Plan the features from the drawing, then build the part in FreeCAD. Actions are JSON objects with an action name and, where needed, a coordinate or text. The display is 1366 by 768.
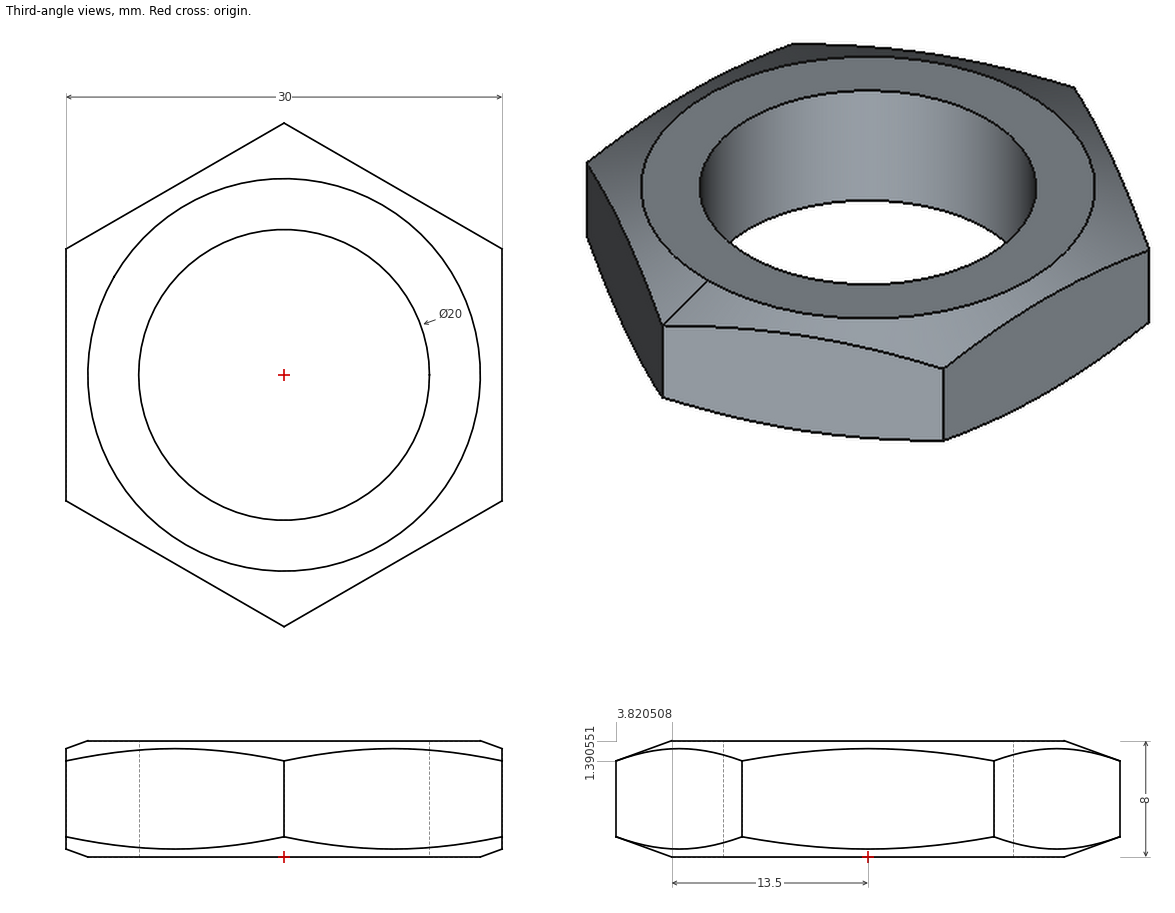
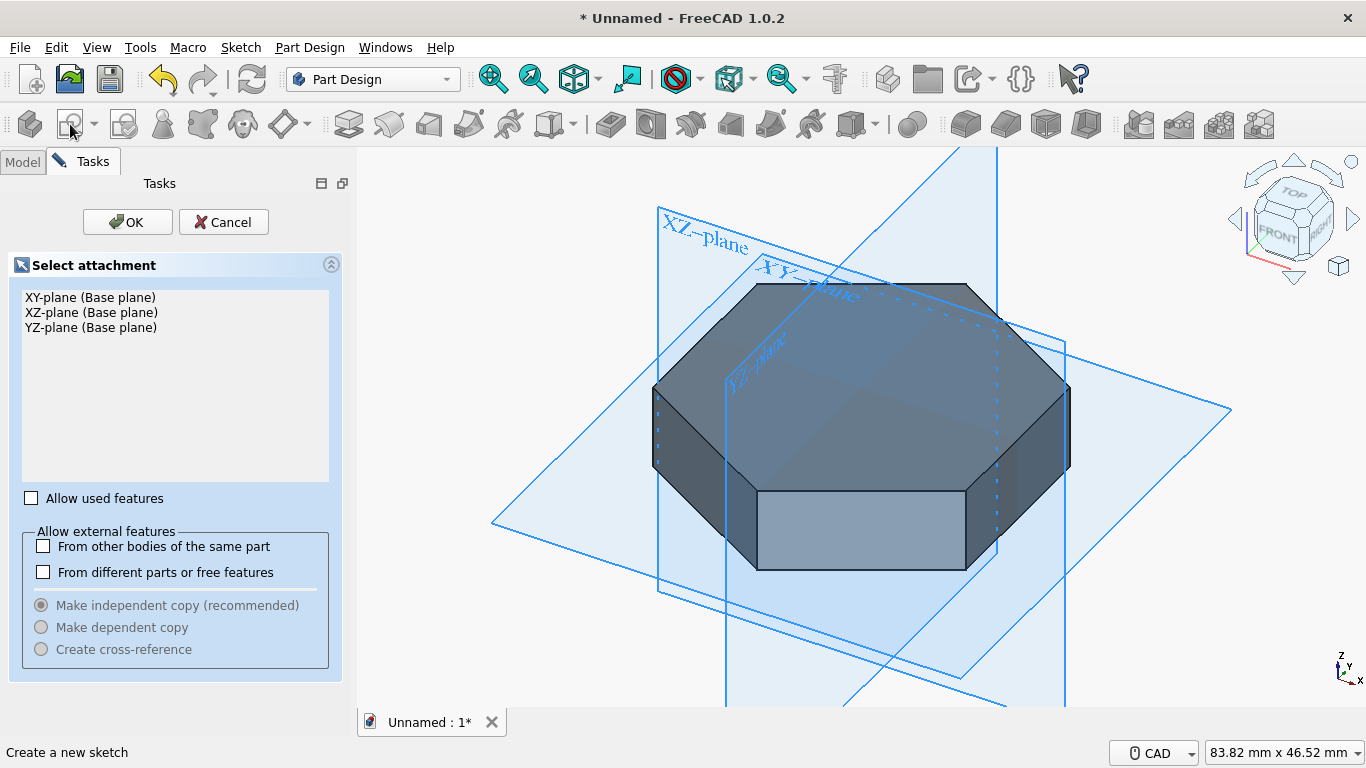
{"action": "left_click", "coordinate": [82, 328]}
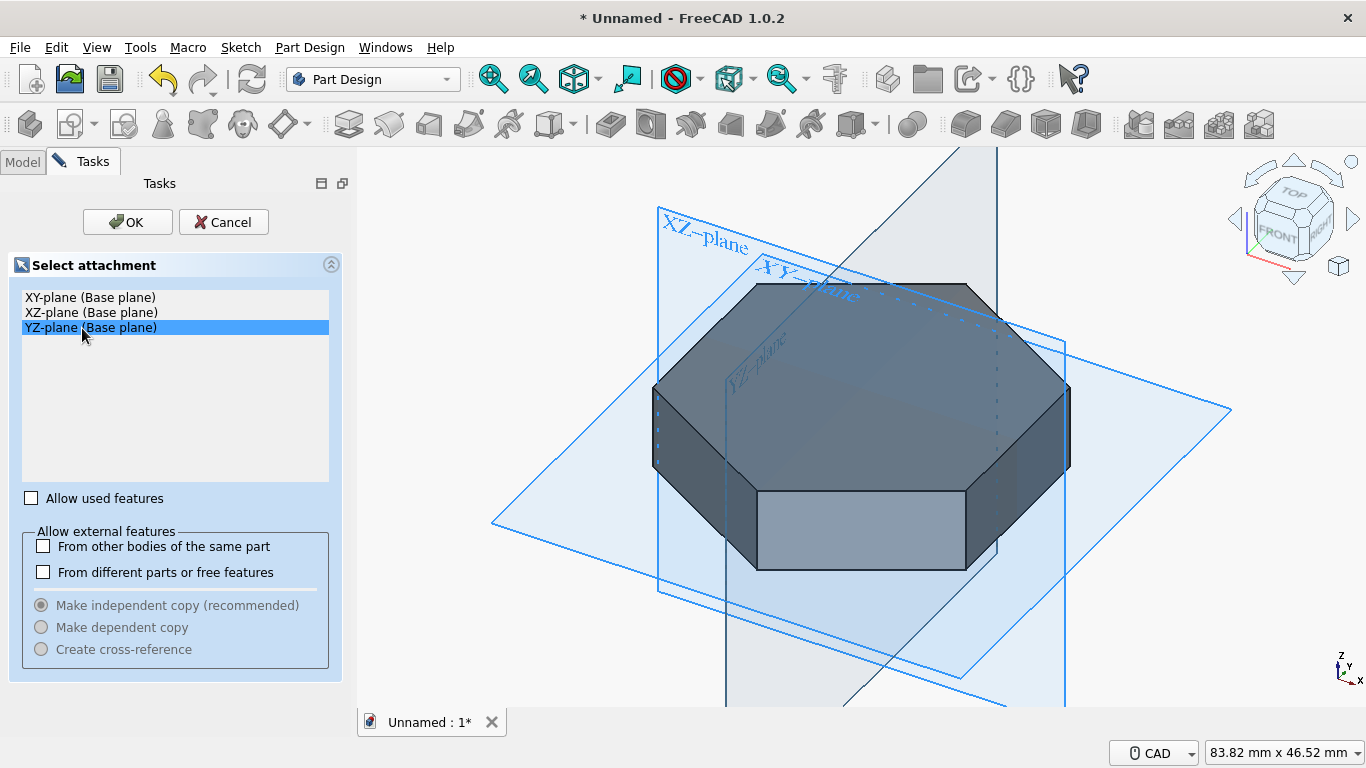
{"action": "left_click", "coordinate": [128, 222]}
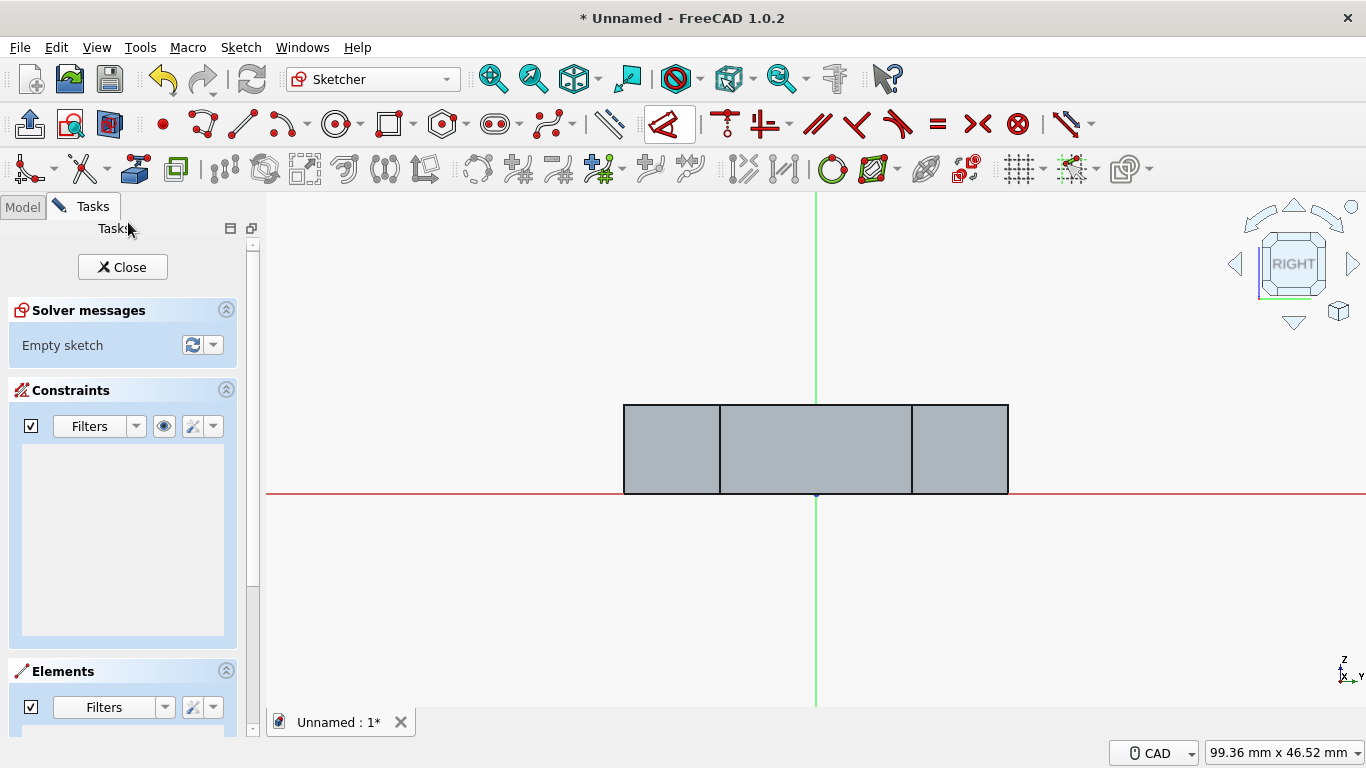
{"action": "left_click", "coordinate": [110, 124]}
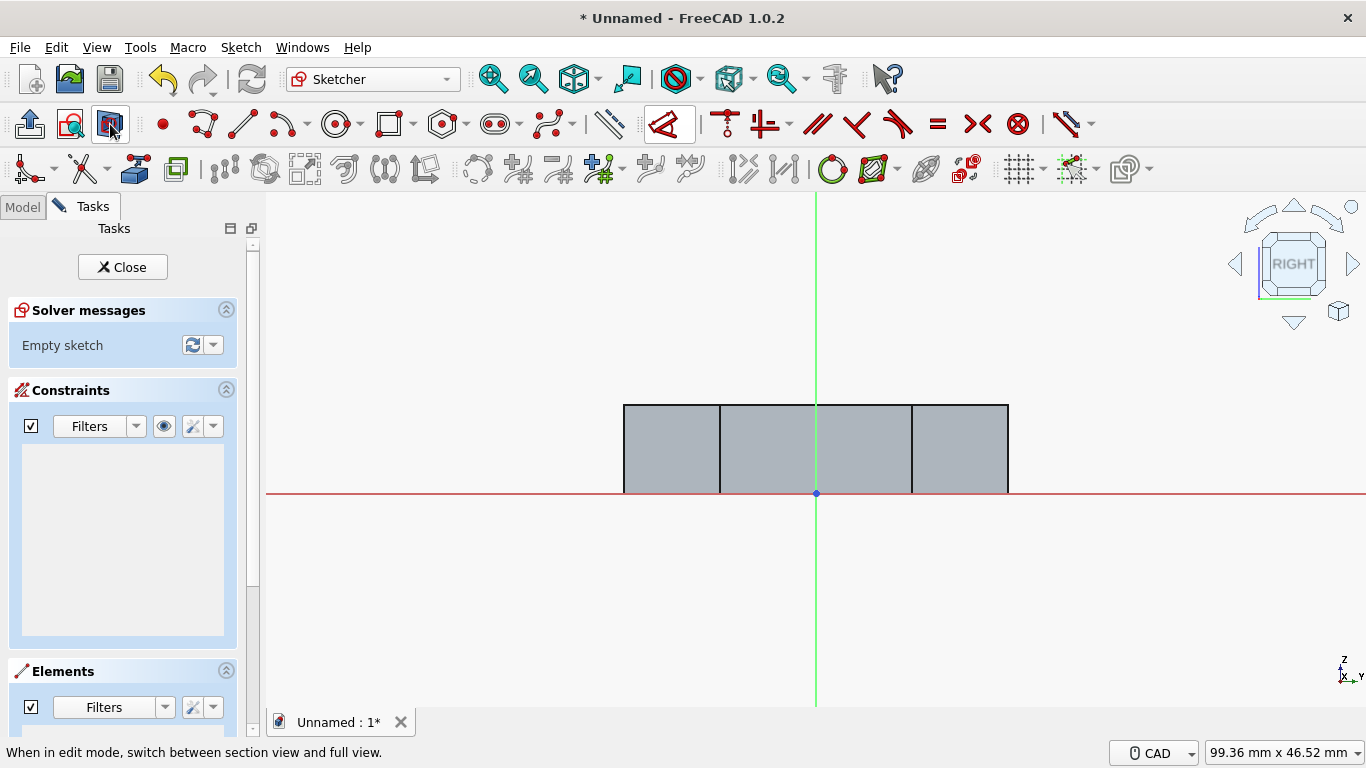
{"action": "scroll", "coordinate": [639, 411], "scroll_direction": "up", "scroll_amount": 14}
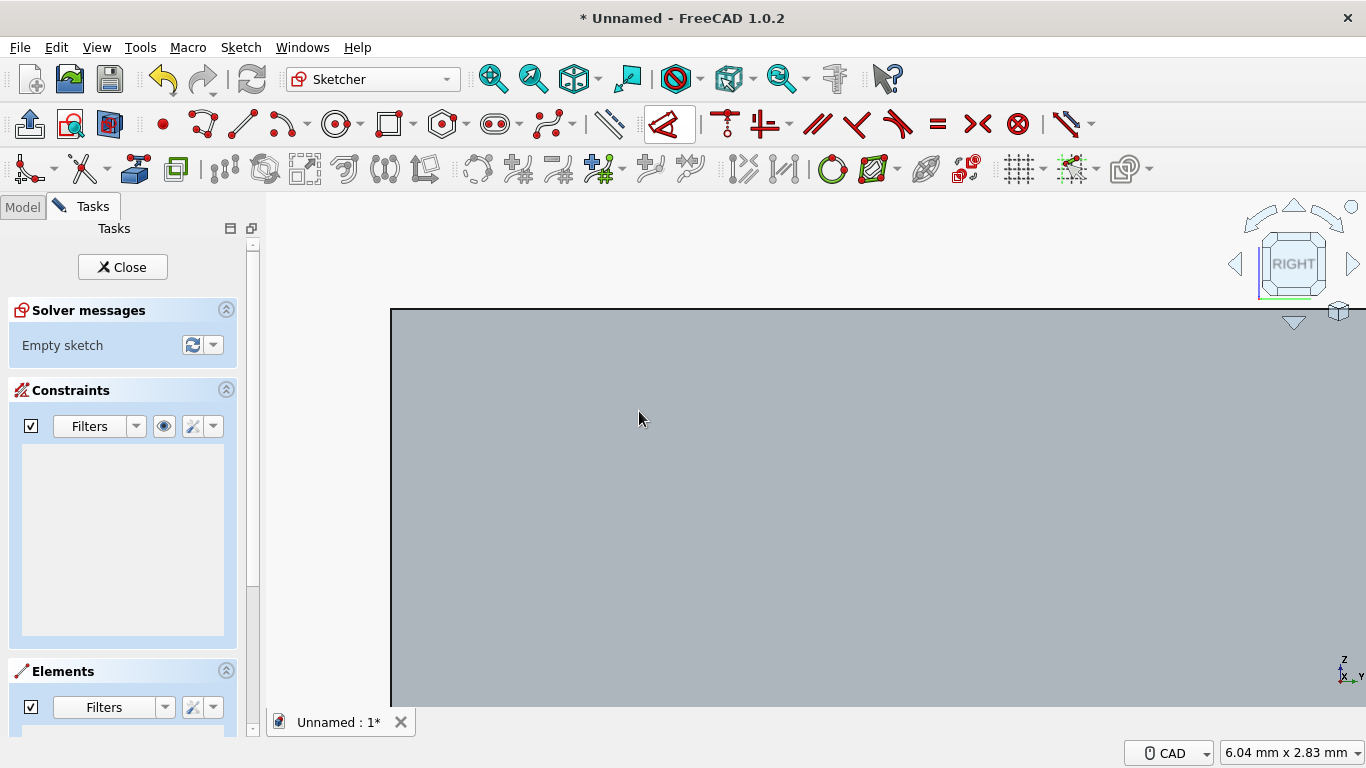
{"action": "left_click", "coordinate": [204, 124]}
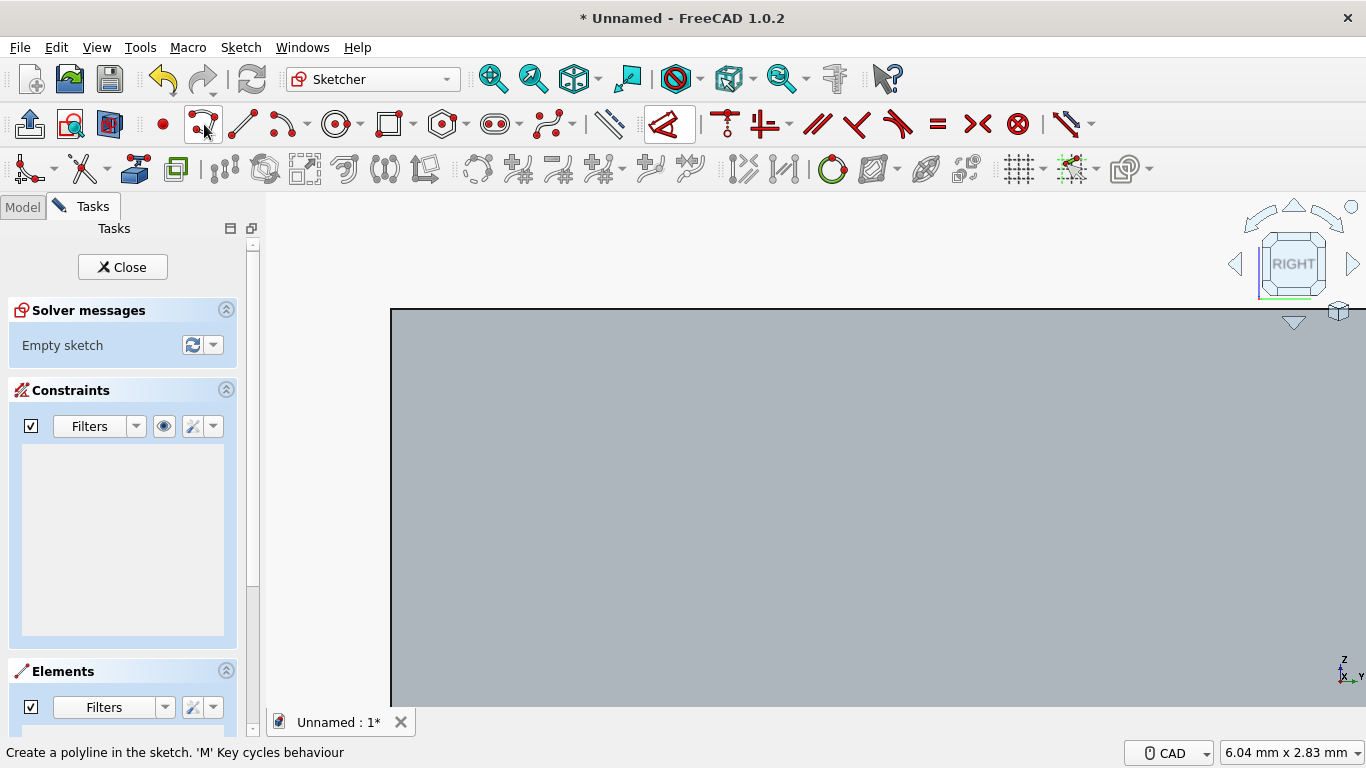
{"action": "left_click", "coordinate": [1087, 309]}
{"action": "left_click", "coordinate": [391, 309]}
{"action": "left_click", "coordinate": [391, 562]}
{"action": "left_click", "coordinate": [1087, 310]}
{"action": "key", "text": "Escape"}
{"action": "key", "text": "Escape"}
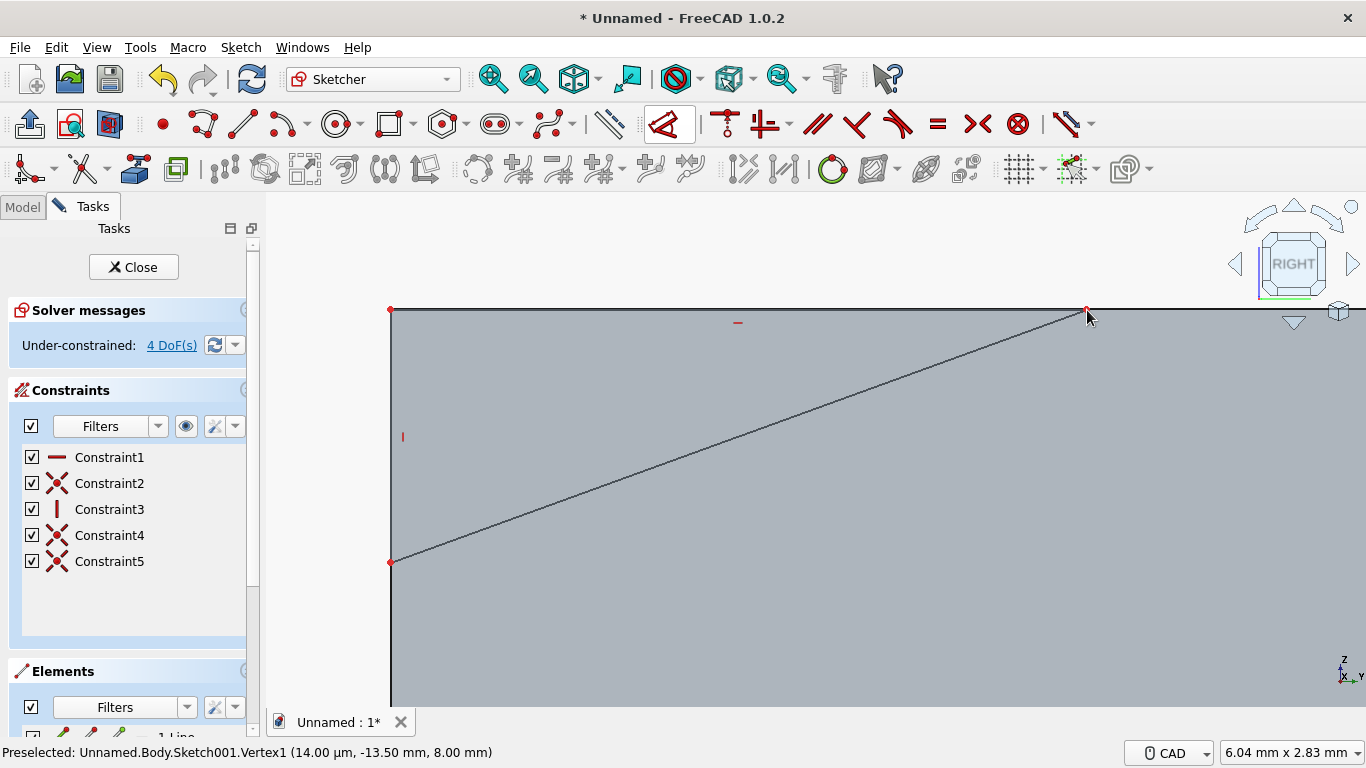
{"action": "key", "text": "d"}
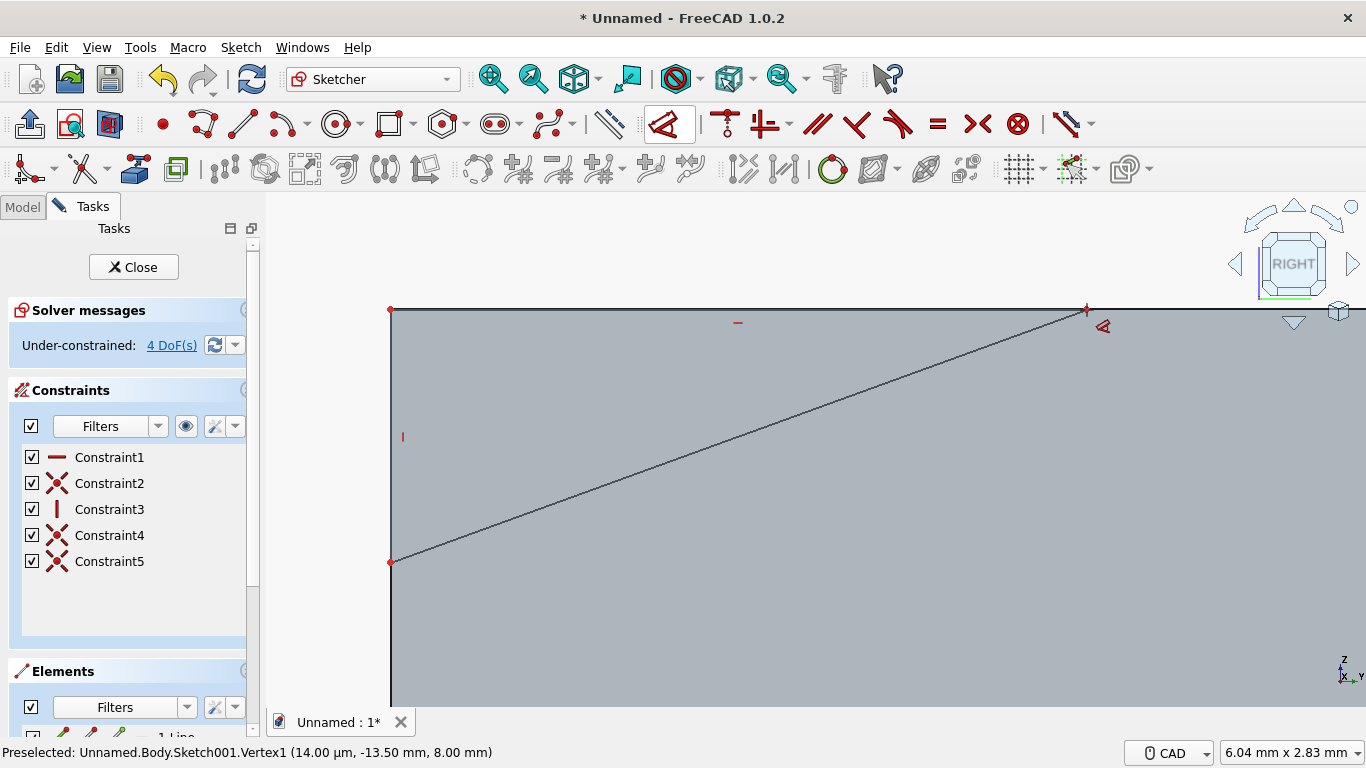
{"action": "left_click", "coordinate": [1087, 310]}
{"action": "left_click", "coordinate": [1053, 494]}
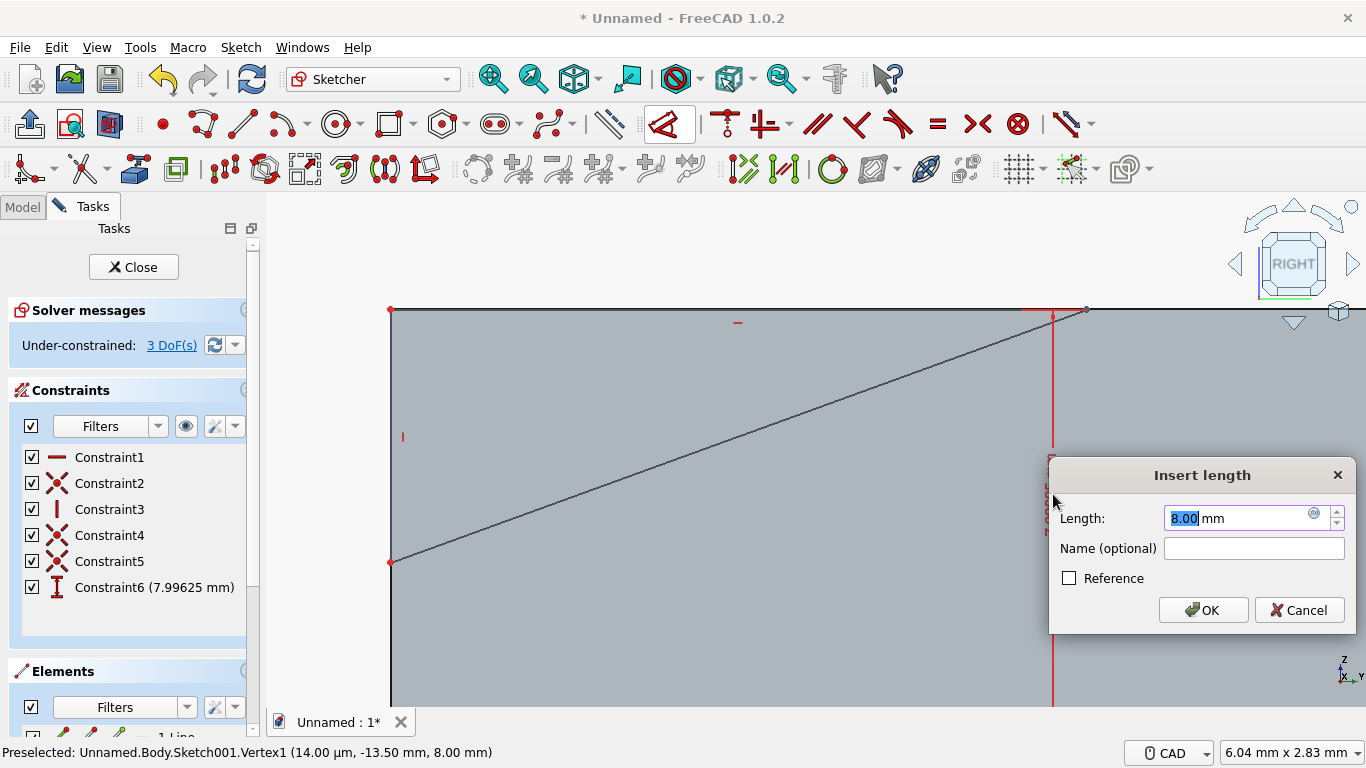
{"action": "type", "text": "8"}
{"action": "key", "text": "Return"}